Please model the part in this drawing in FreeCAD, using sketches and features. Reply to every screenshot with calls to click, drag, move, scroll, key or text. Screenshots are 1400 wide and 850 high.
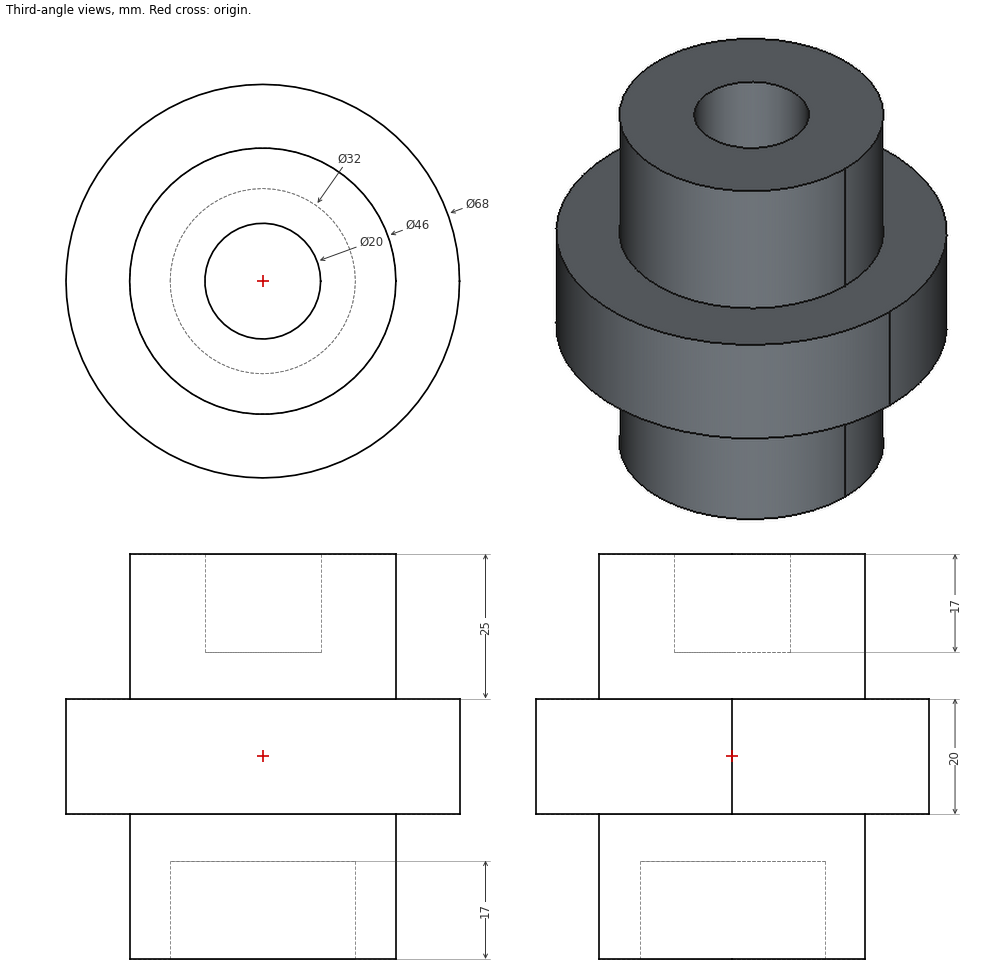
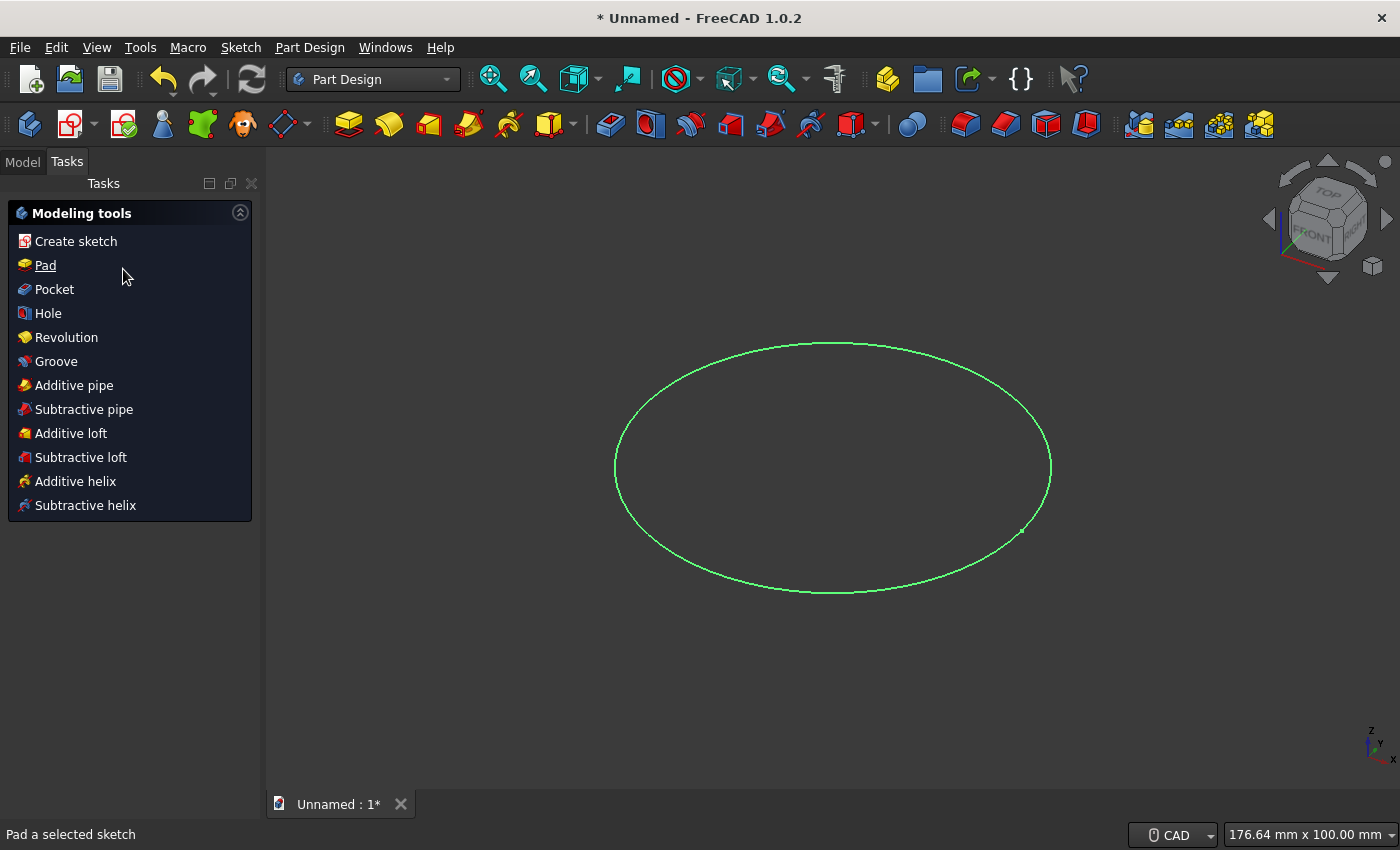
click(350, 124)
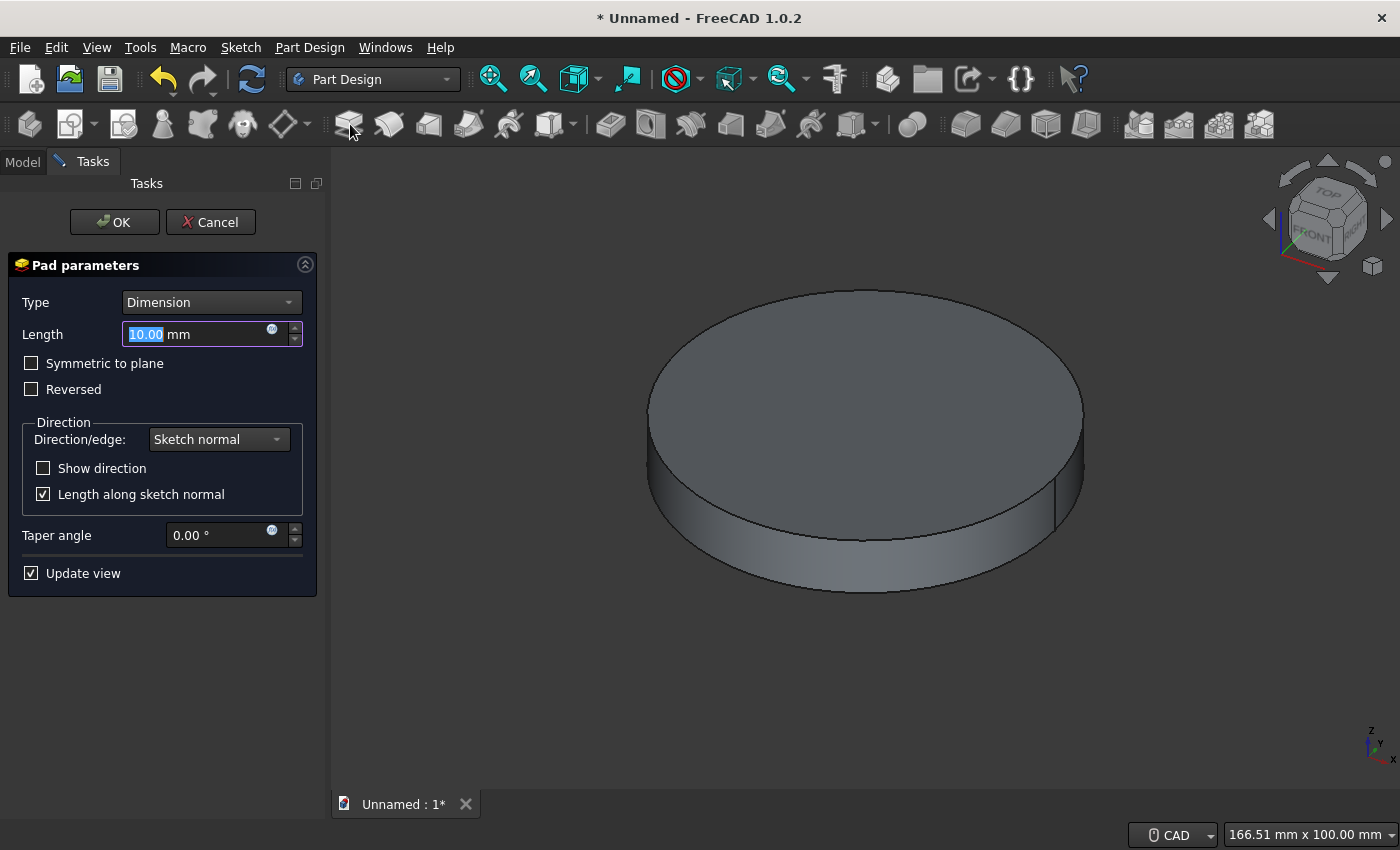
text(20)
key(Tab)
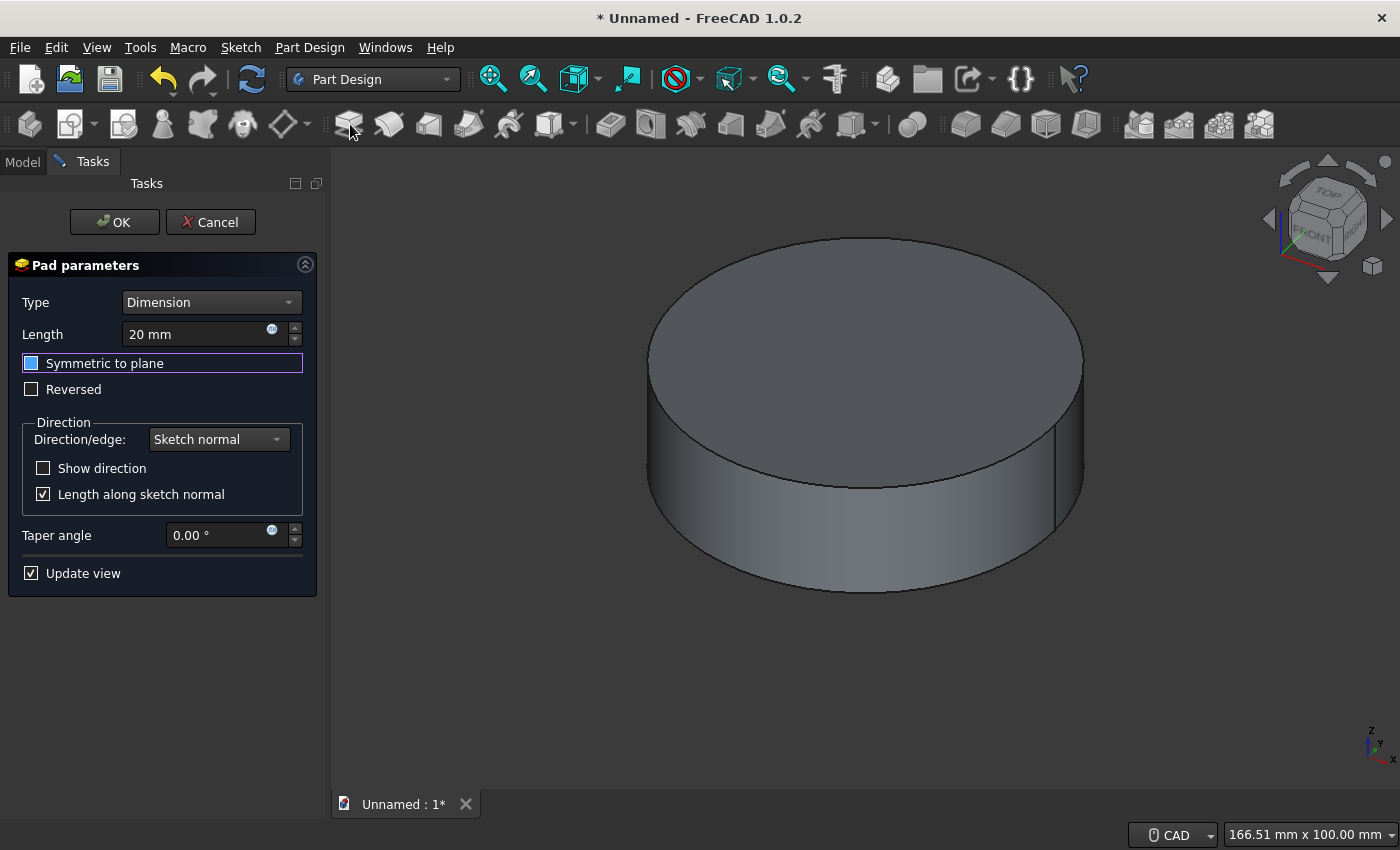
click(30, 363)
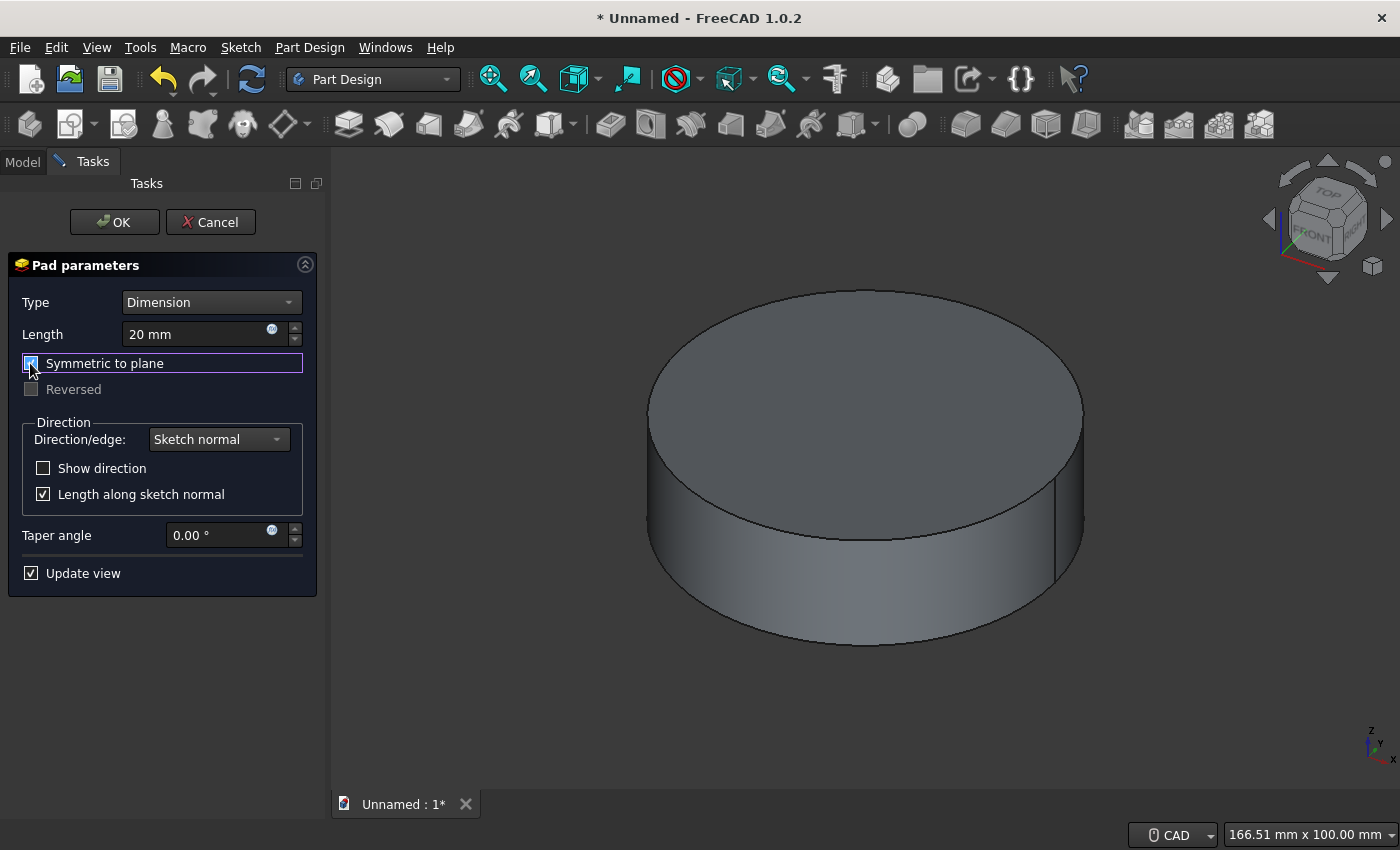
click(115, 222)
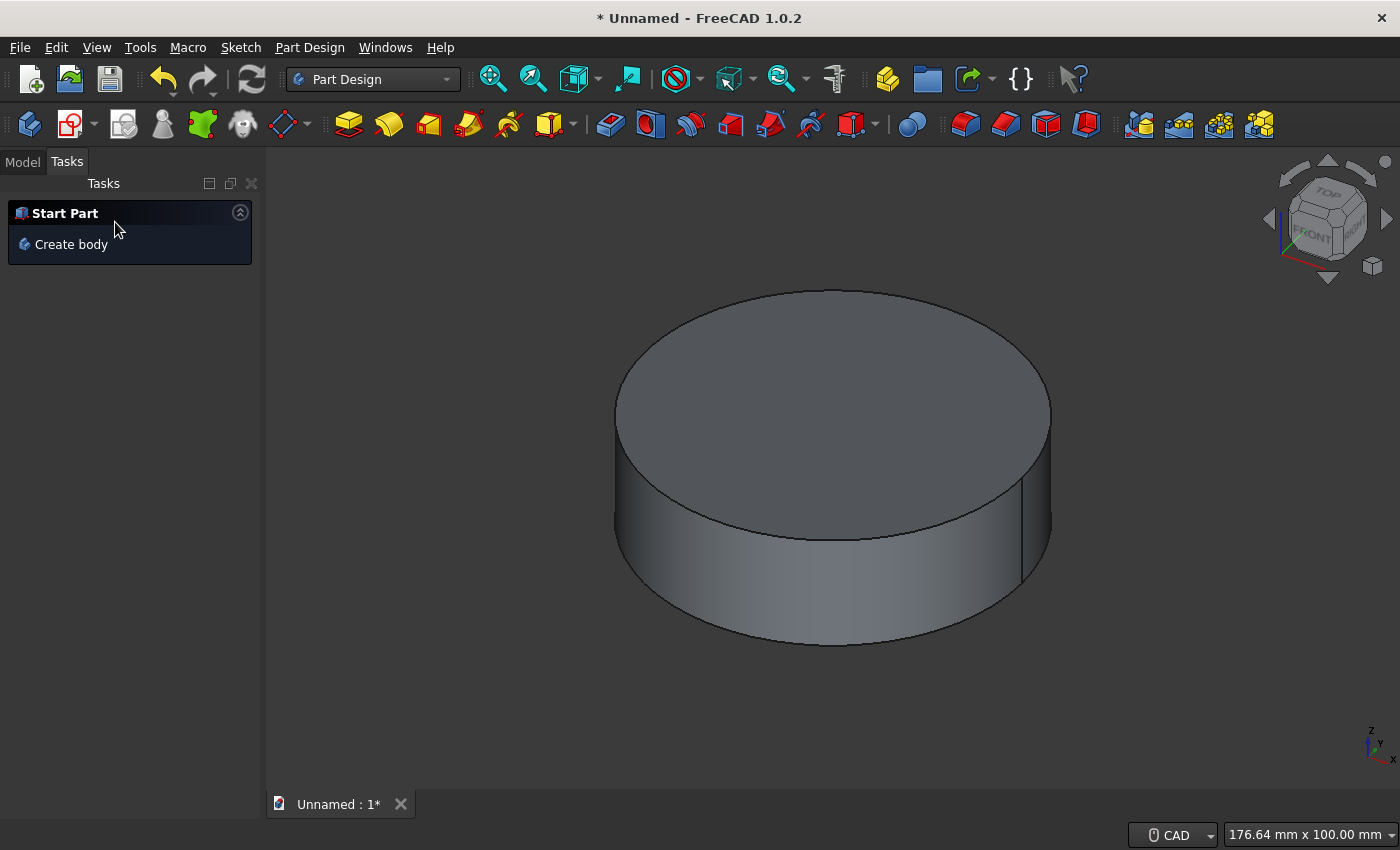
click(833, 414)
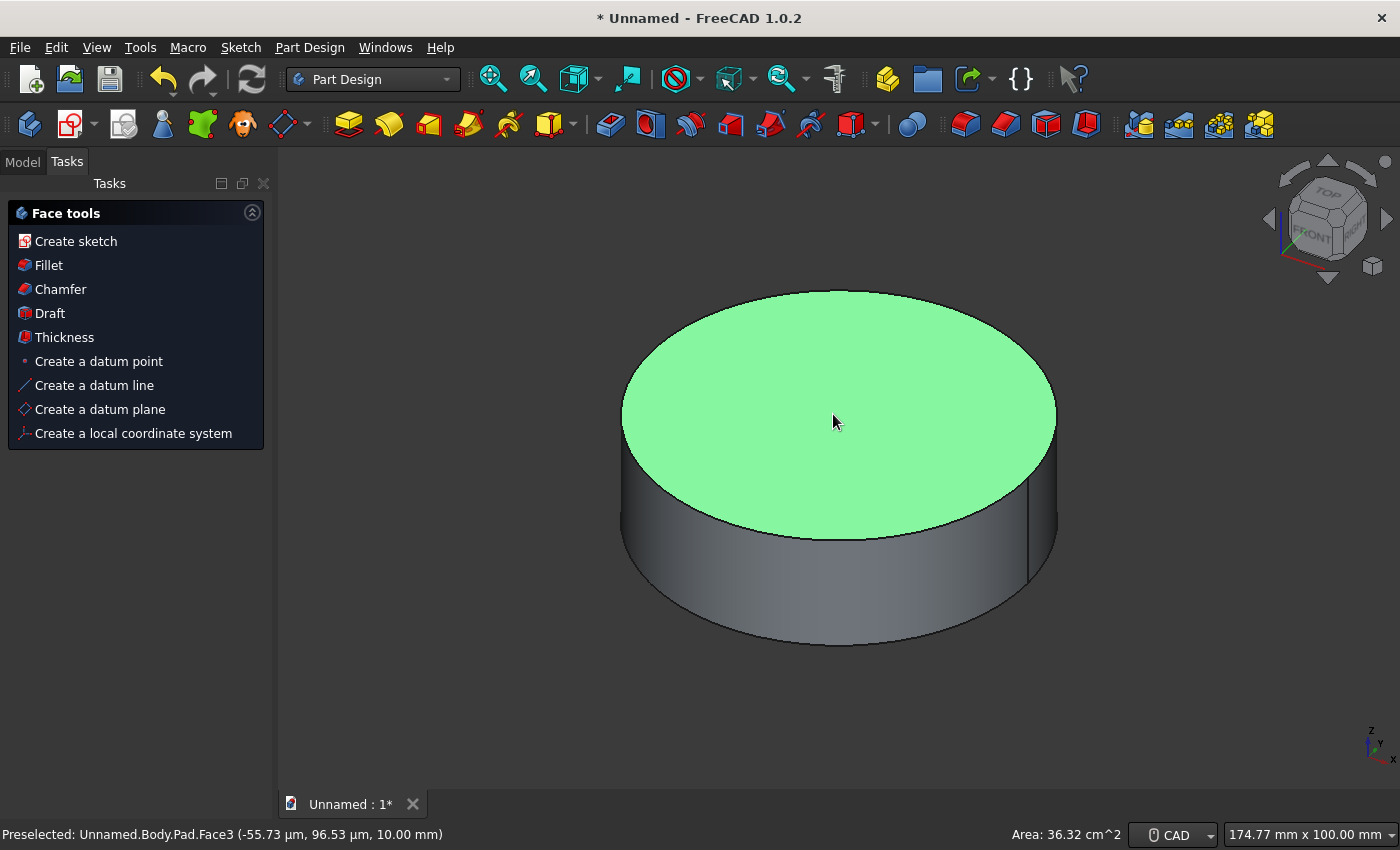
click(70, 124)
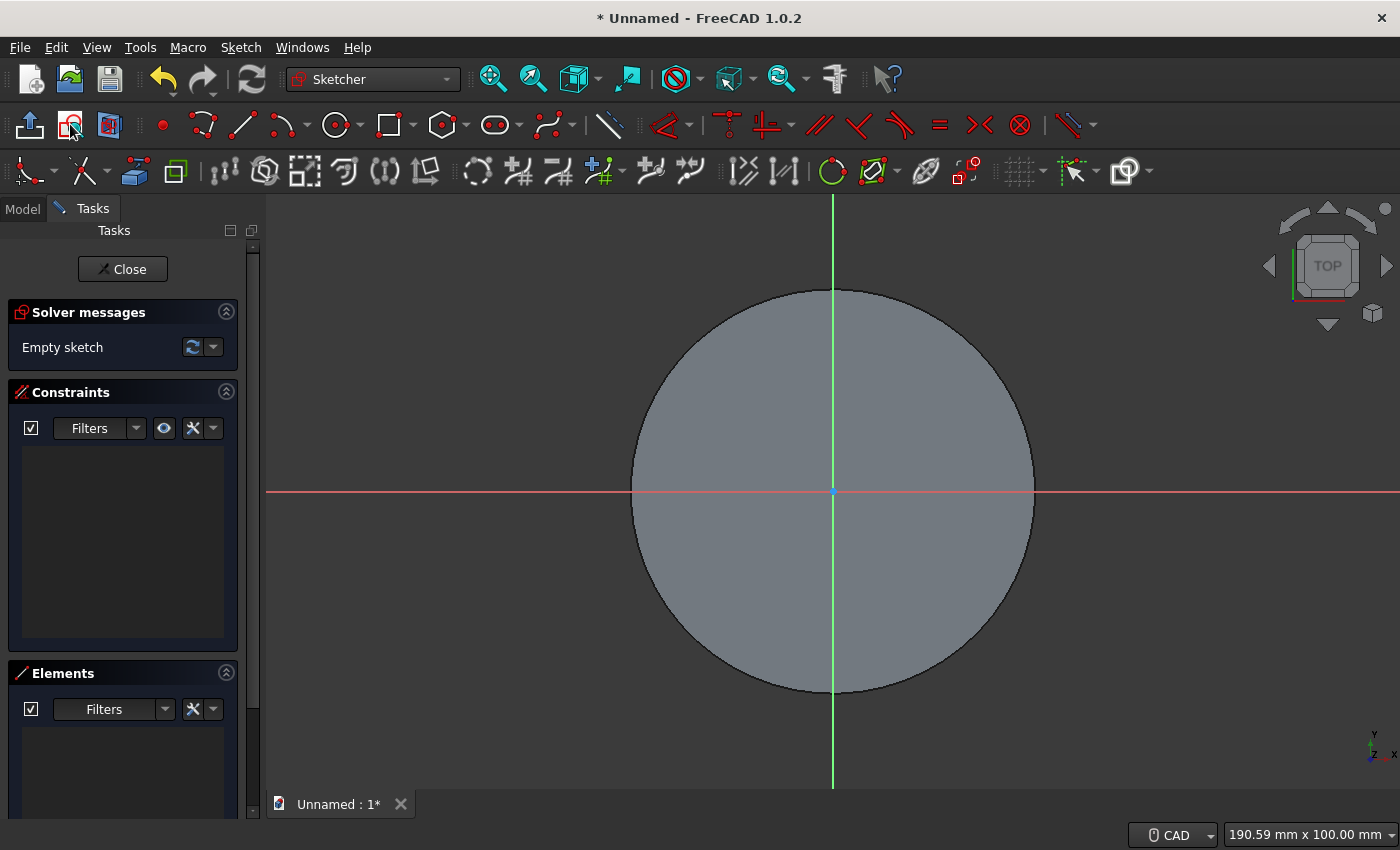
scroll(972, 491, up, 2)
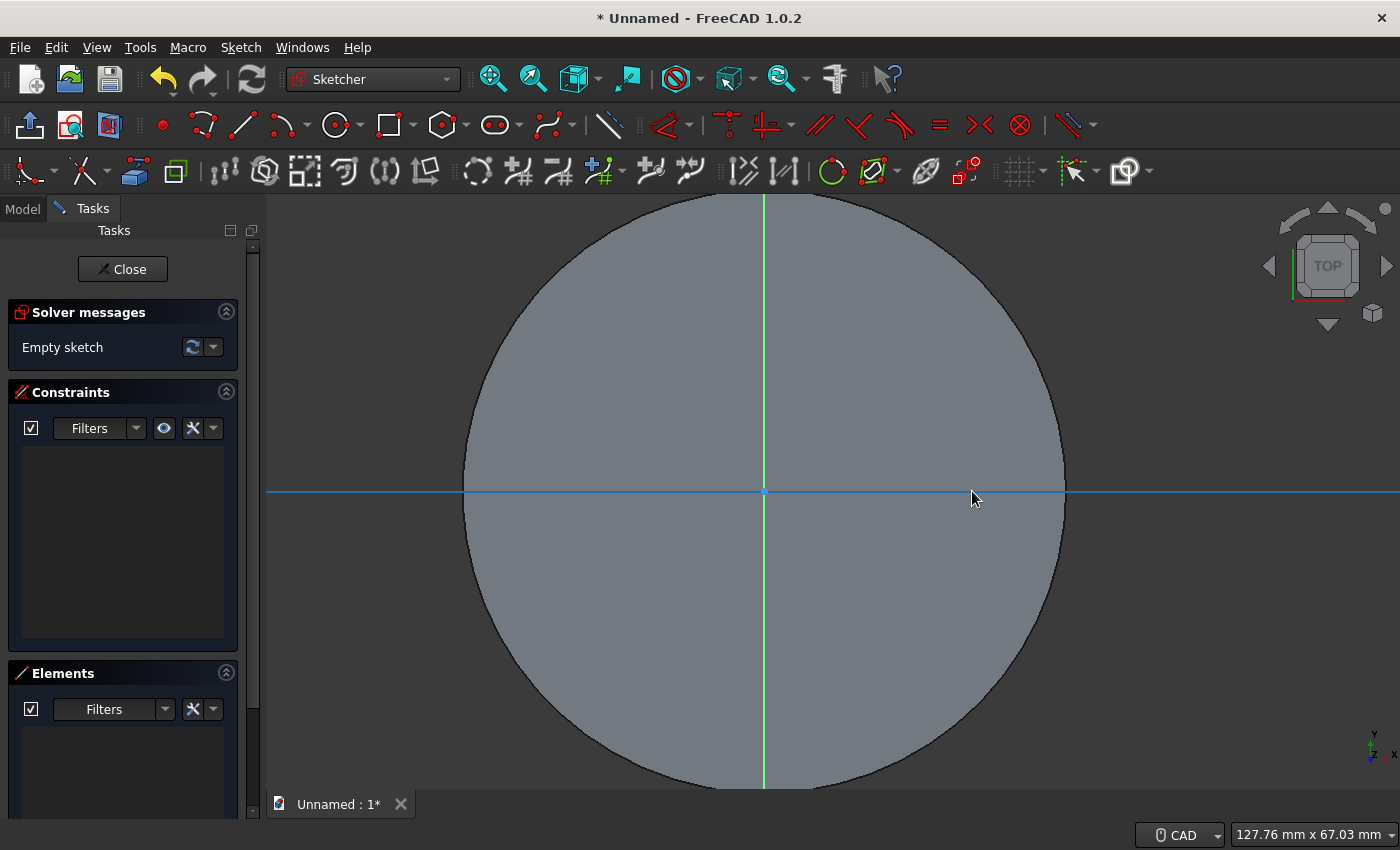
click(336, 126)